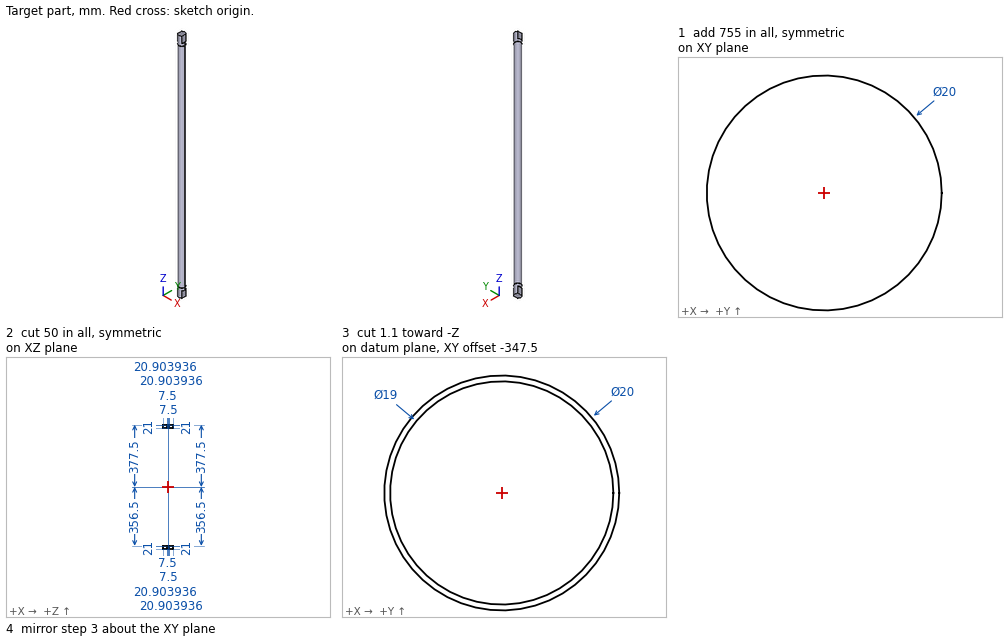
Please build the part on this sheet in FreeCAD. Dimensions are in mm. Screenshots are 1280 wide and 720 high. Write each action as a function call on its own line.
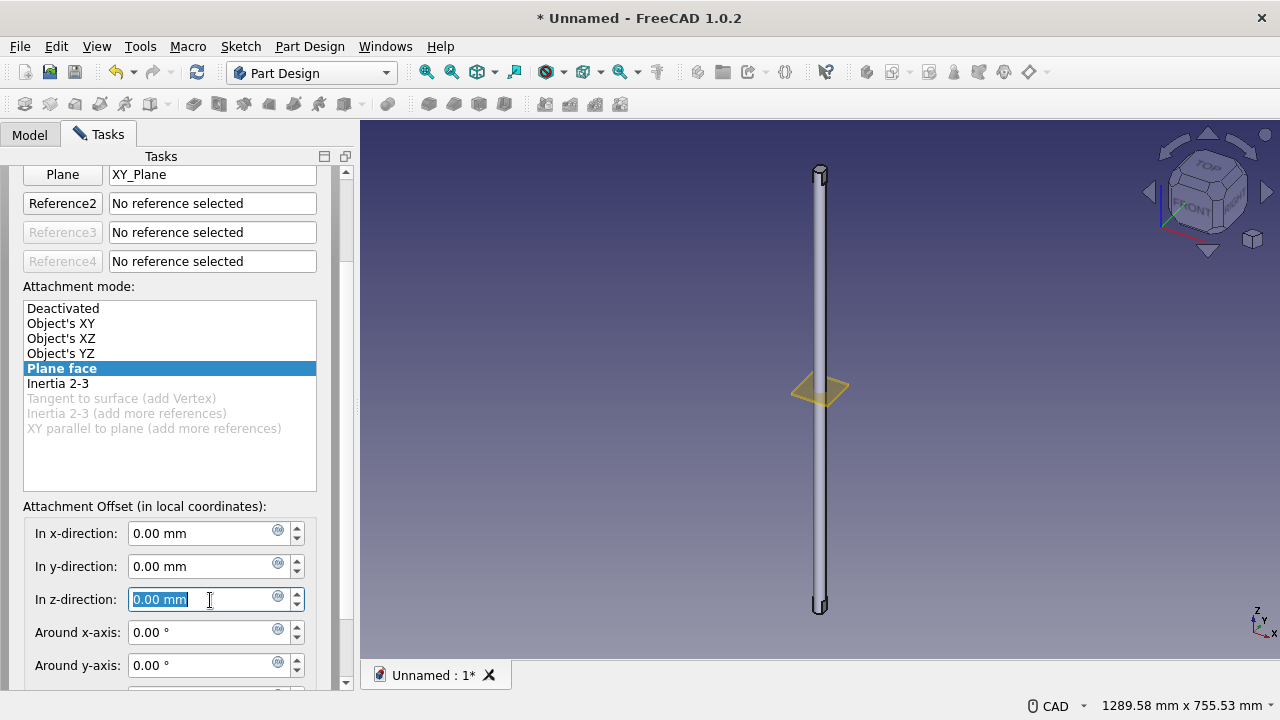
text(-347.5)
key(Tab)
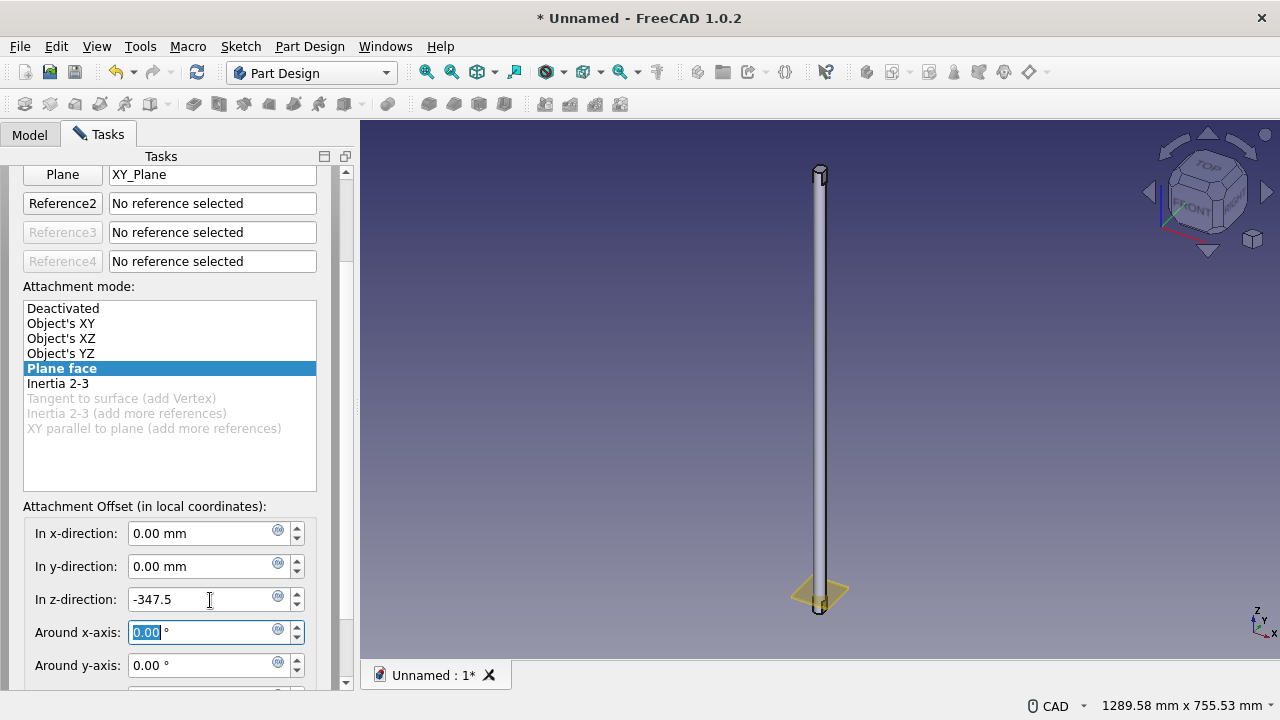
scroll(346, 428, up, 3)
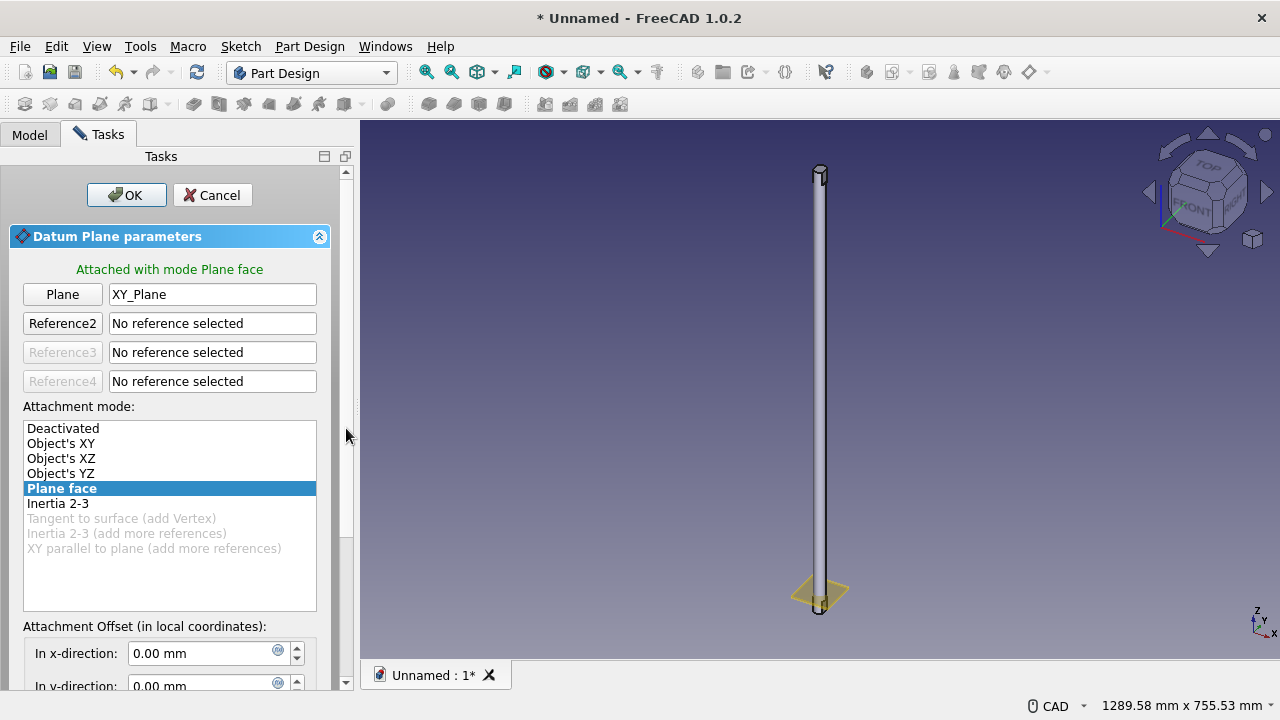
click(127, 195)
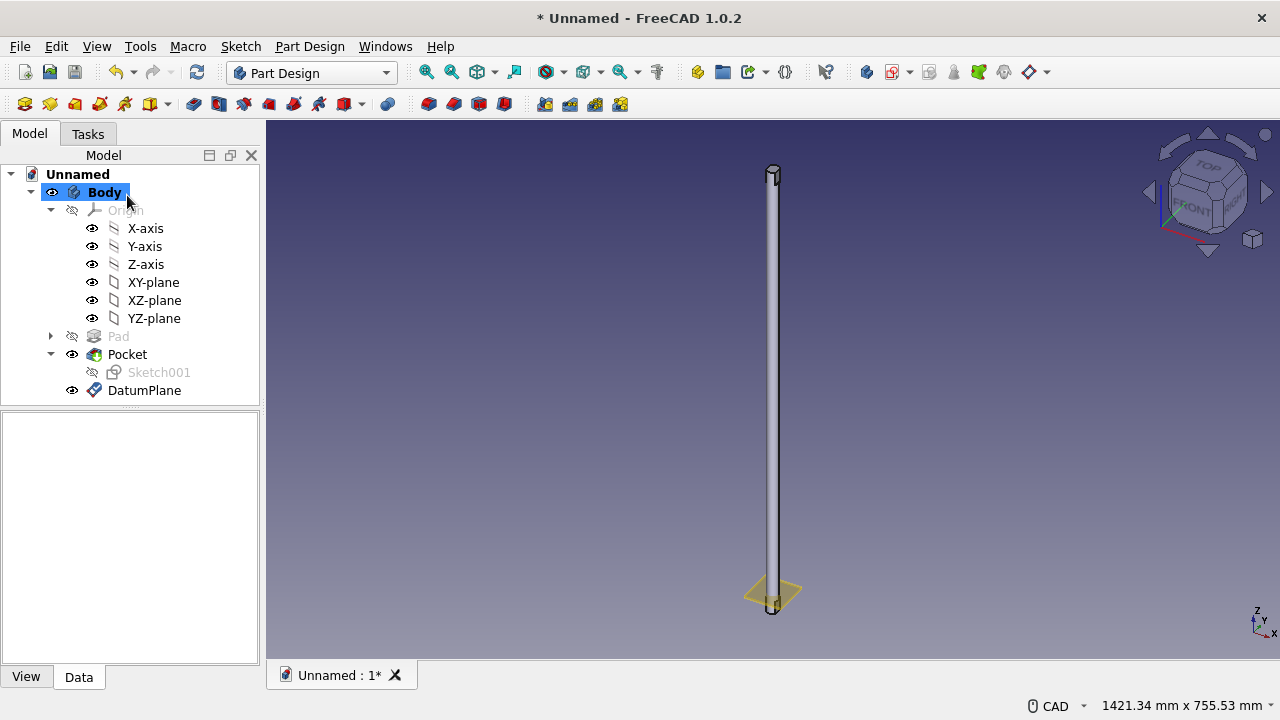
click(117, 390)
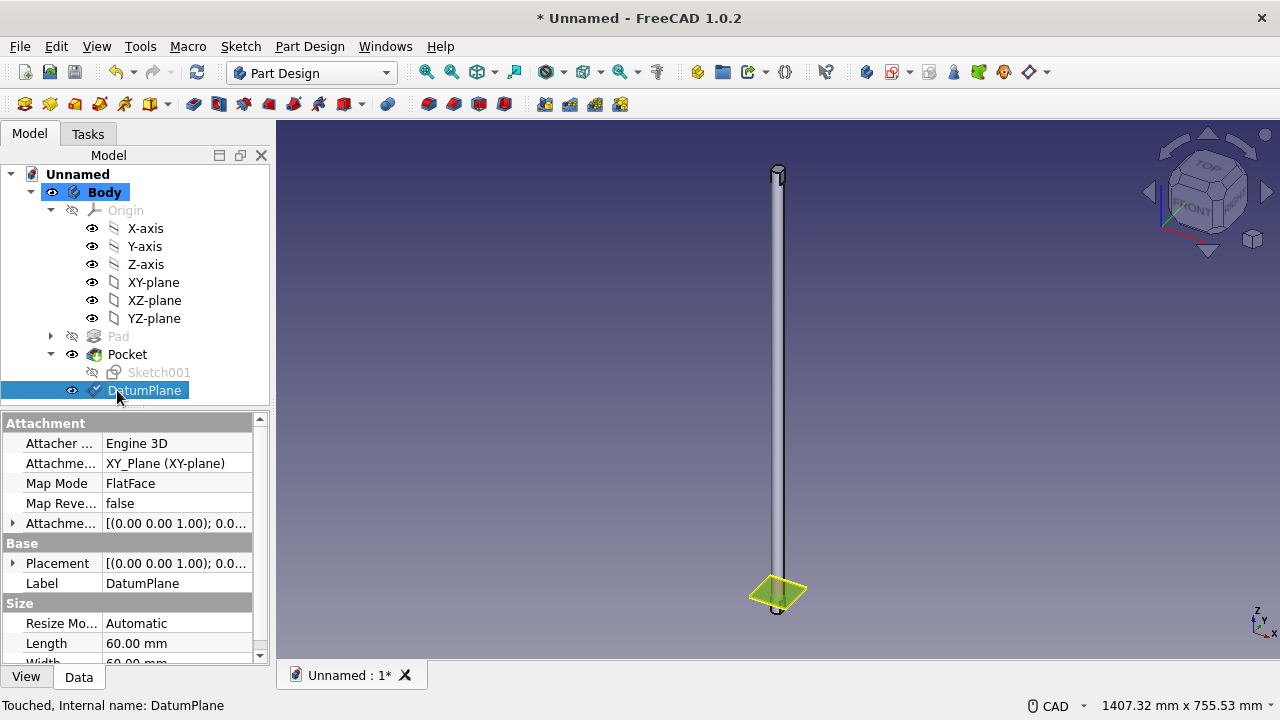
click(892, 72)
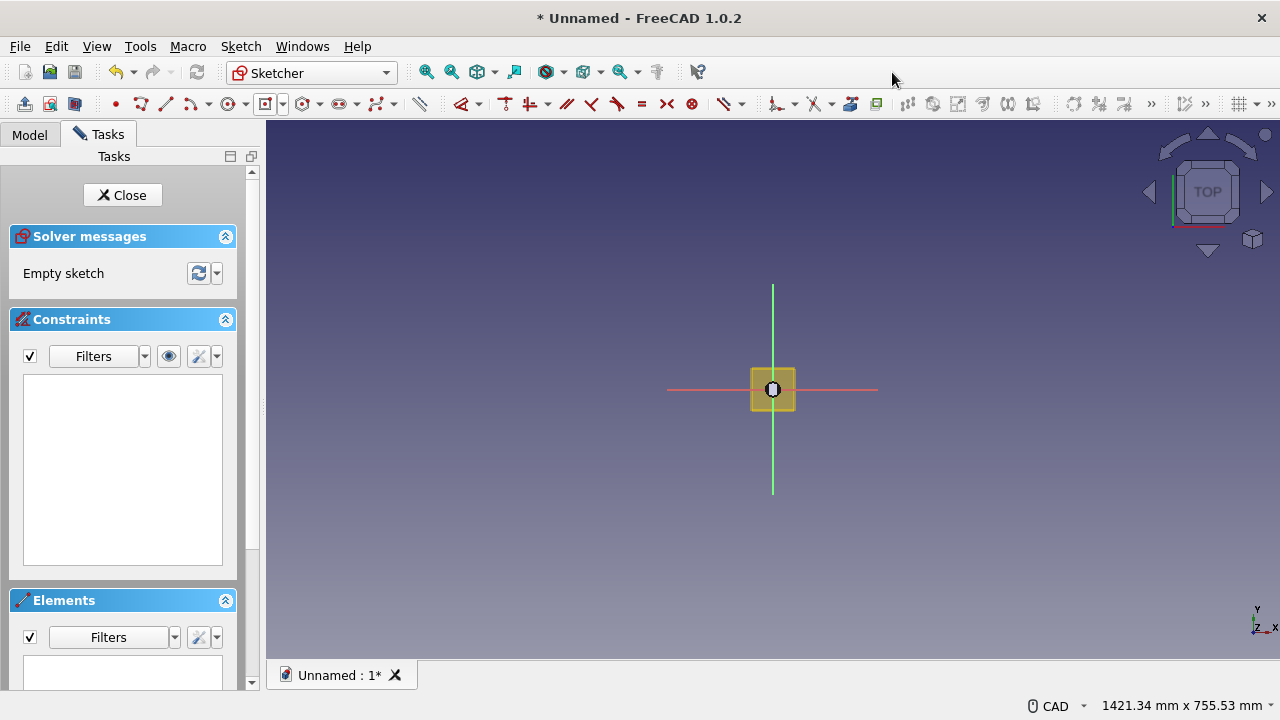
key(q)
key(s)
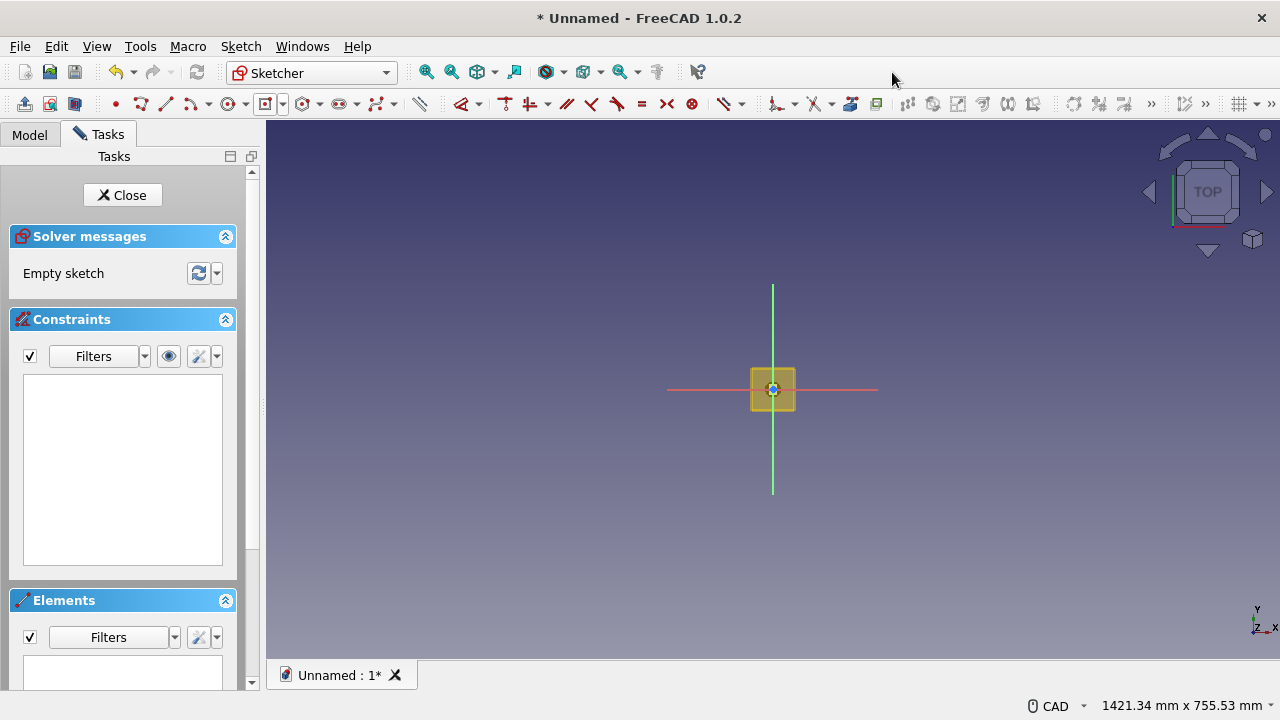
scroll(777, 390, up, 15)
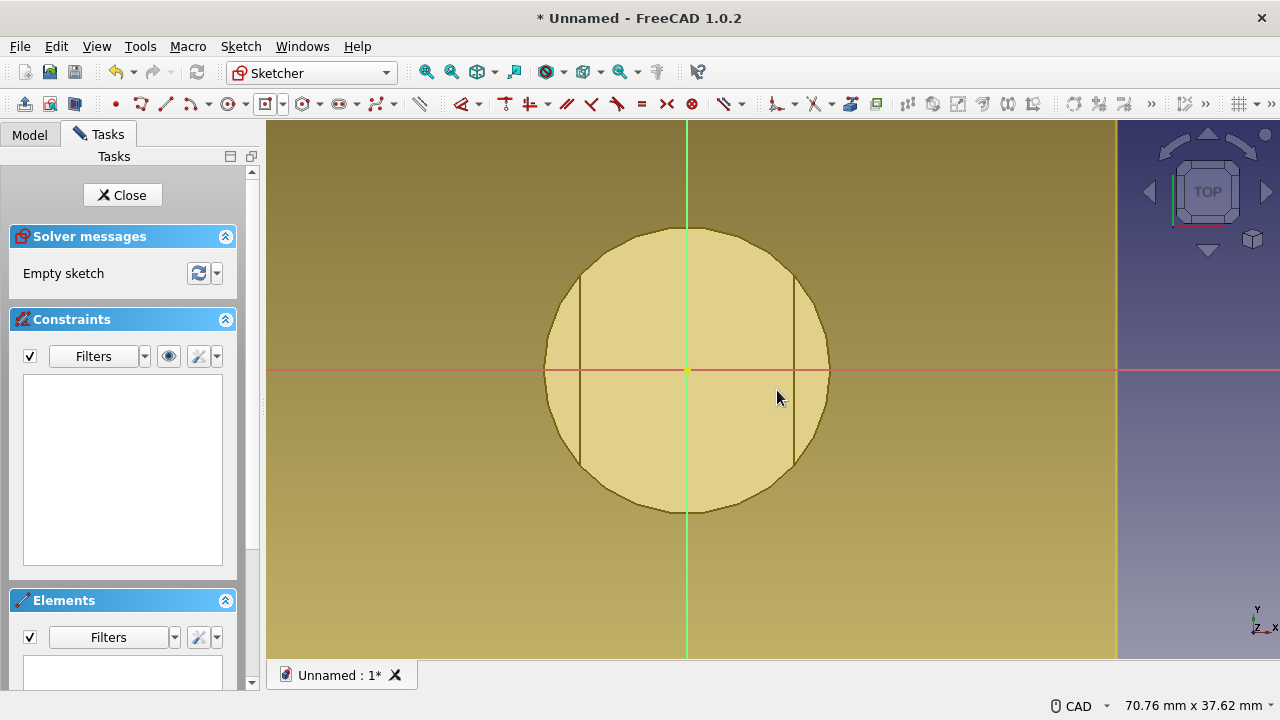
key(g)
key(c)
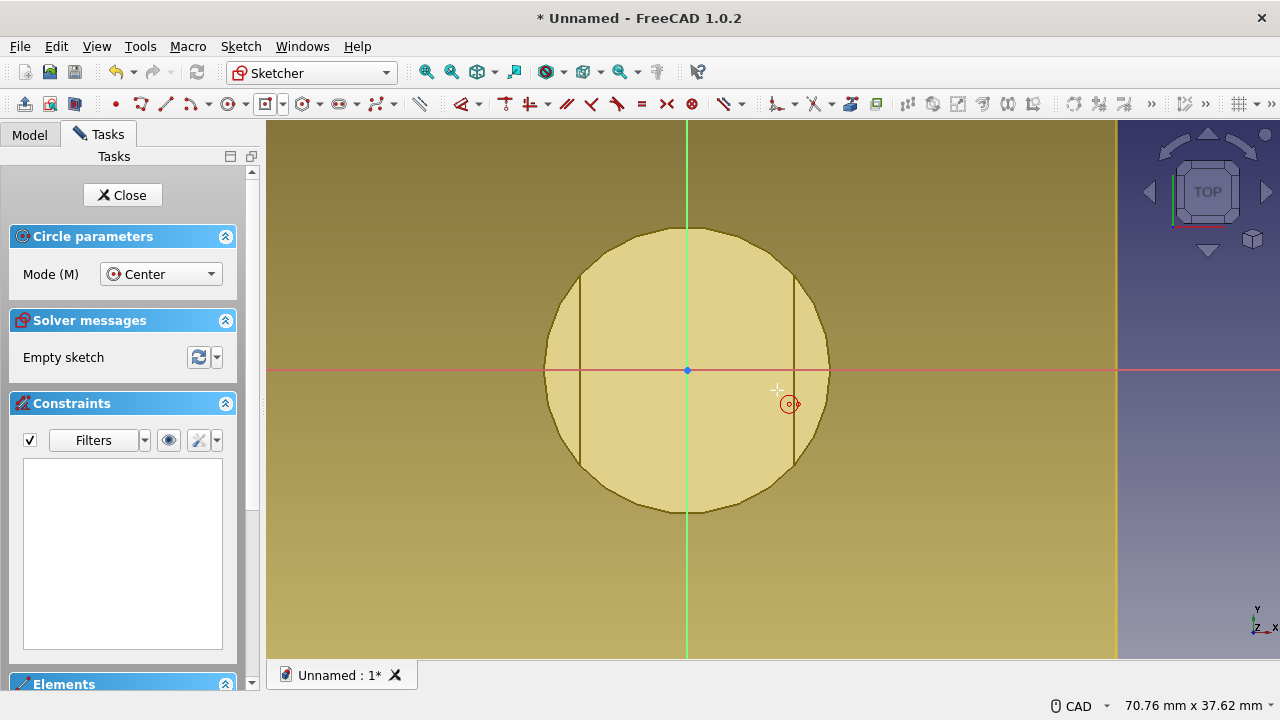
click(687, 370)
move(788, 269)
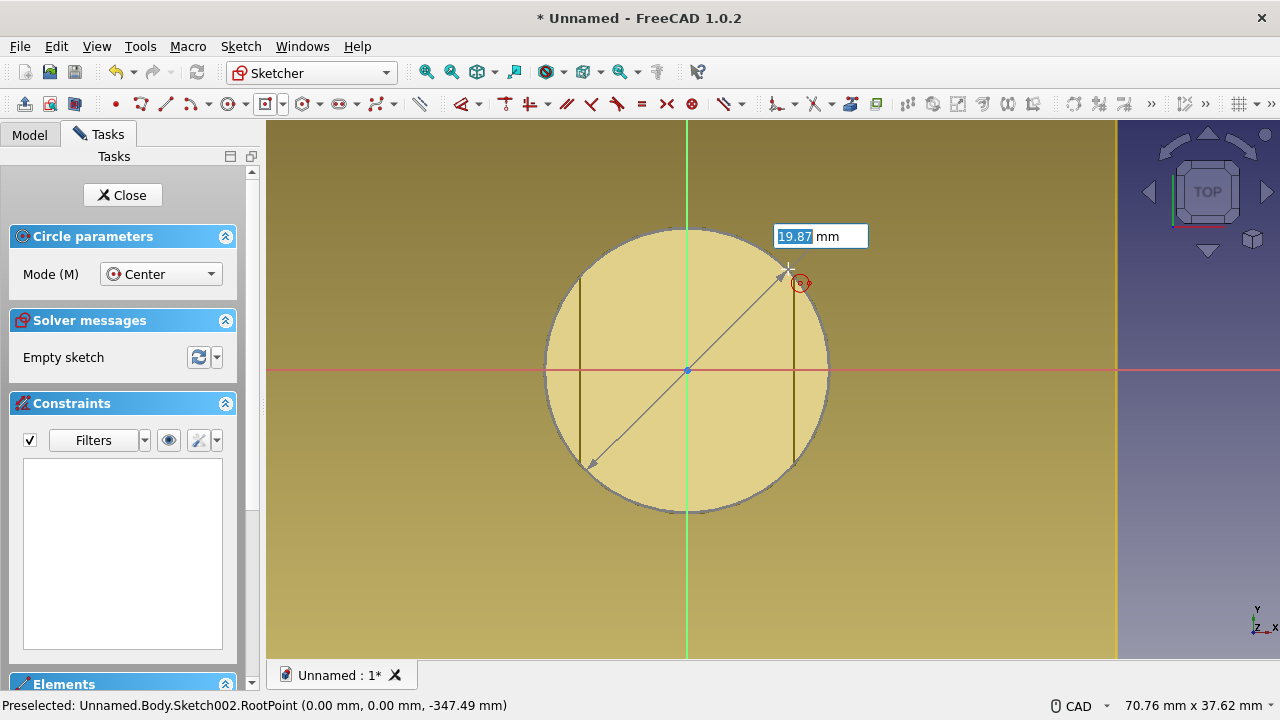
text(20)
key(Return)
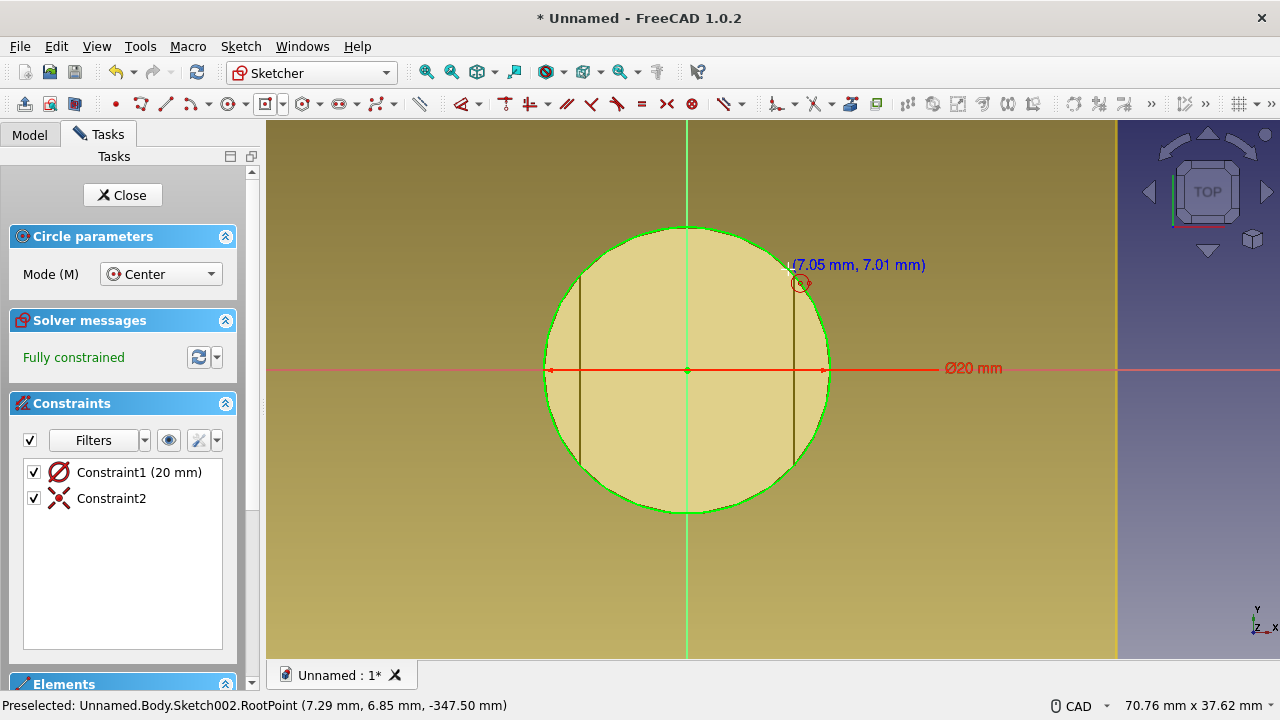
click(687, 370)